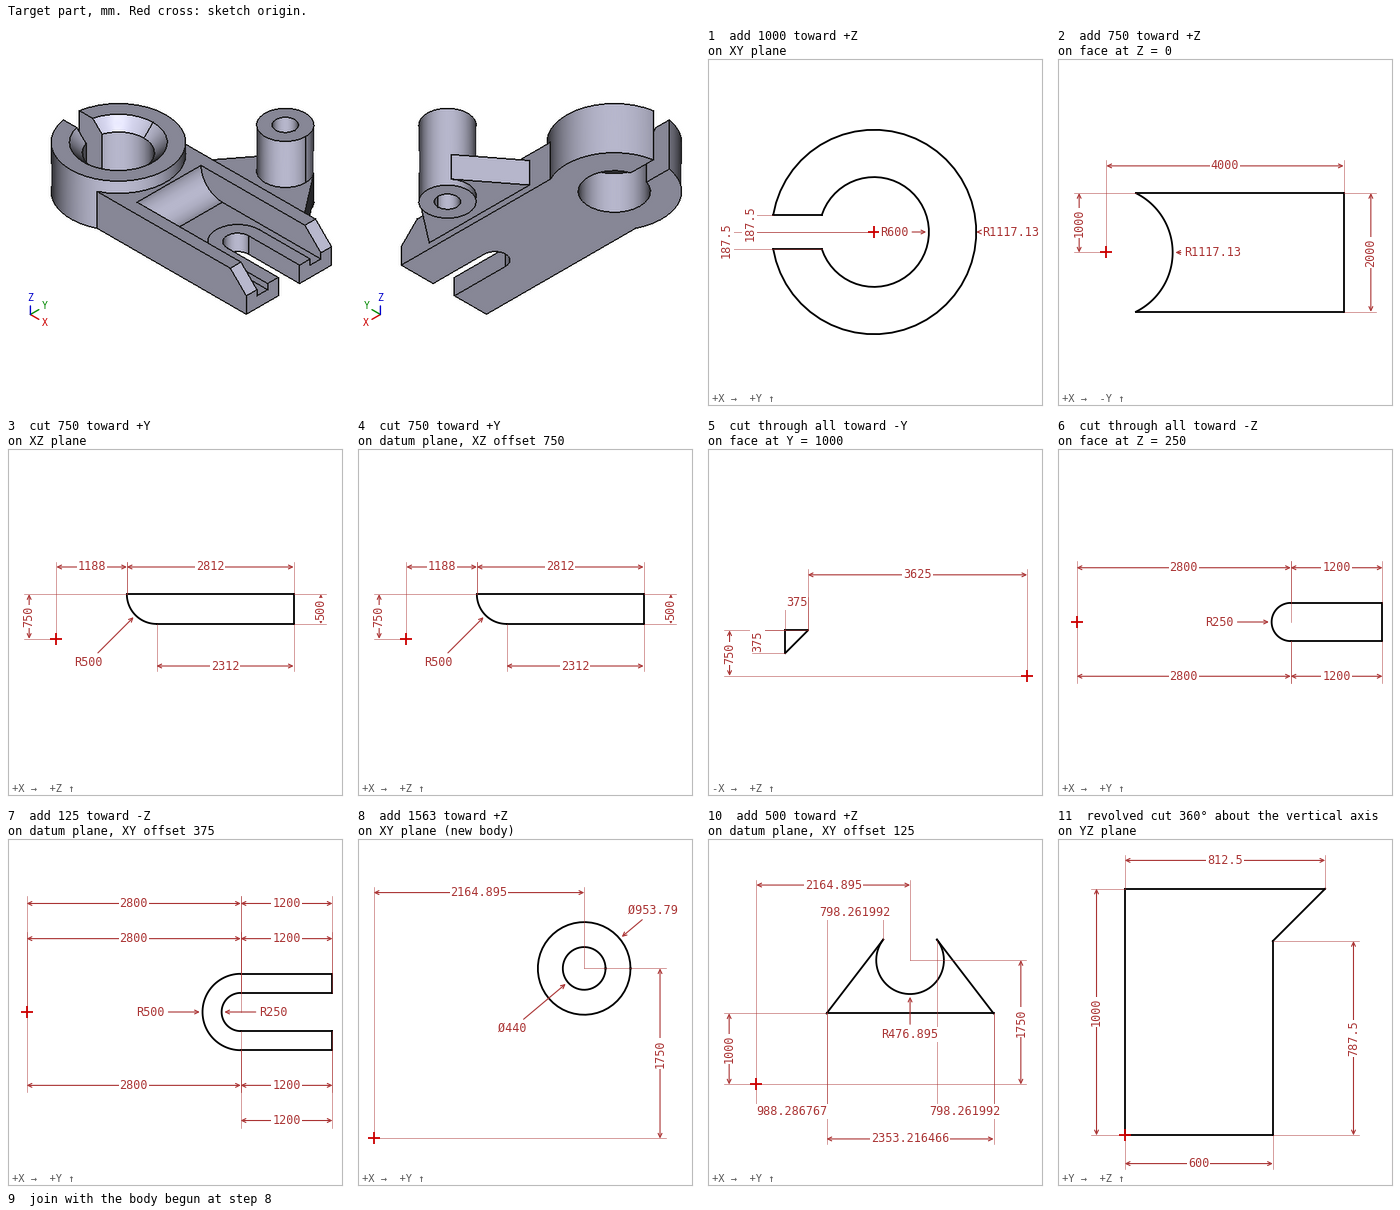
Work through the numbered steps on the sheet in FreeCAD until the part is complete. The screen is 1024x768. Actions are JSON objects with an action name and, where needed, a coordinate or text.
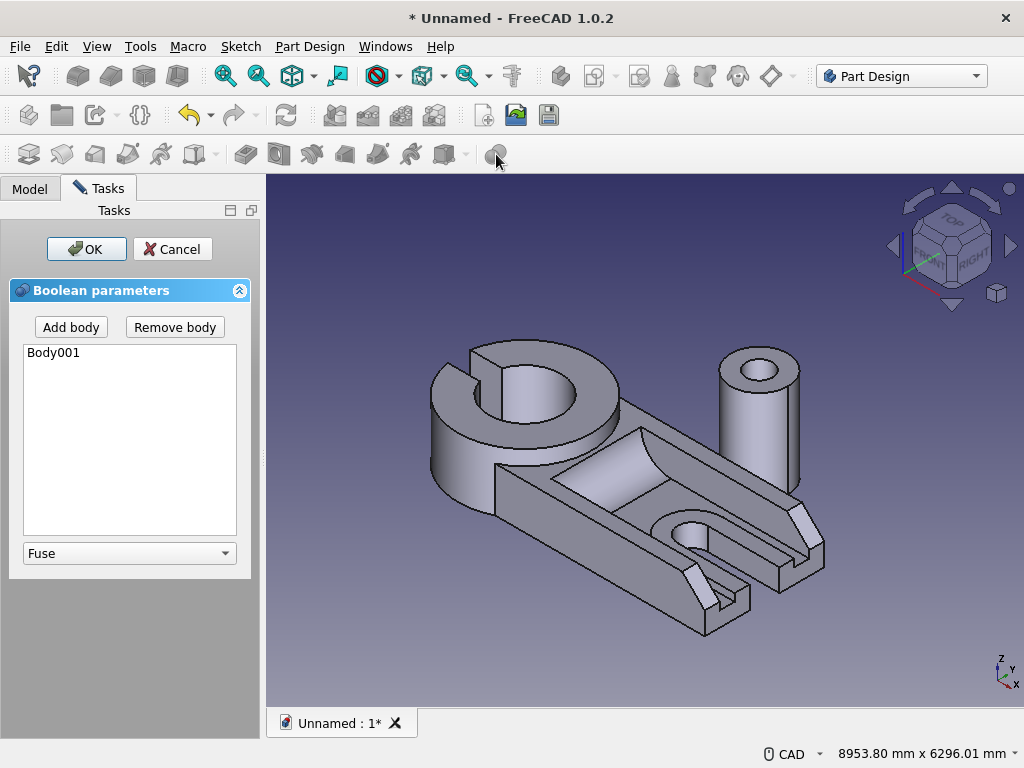
{"action": "left_click", "coordinate": [87, 249]}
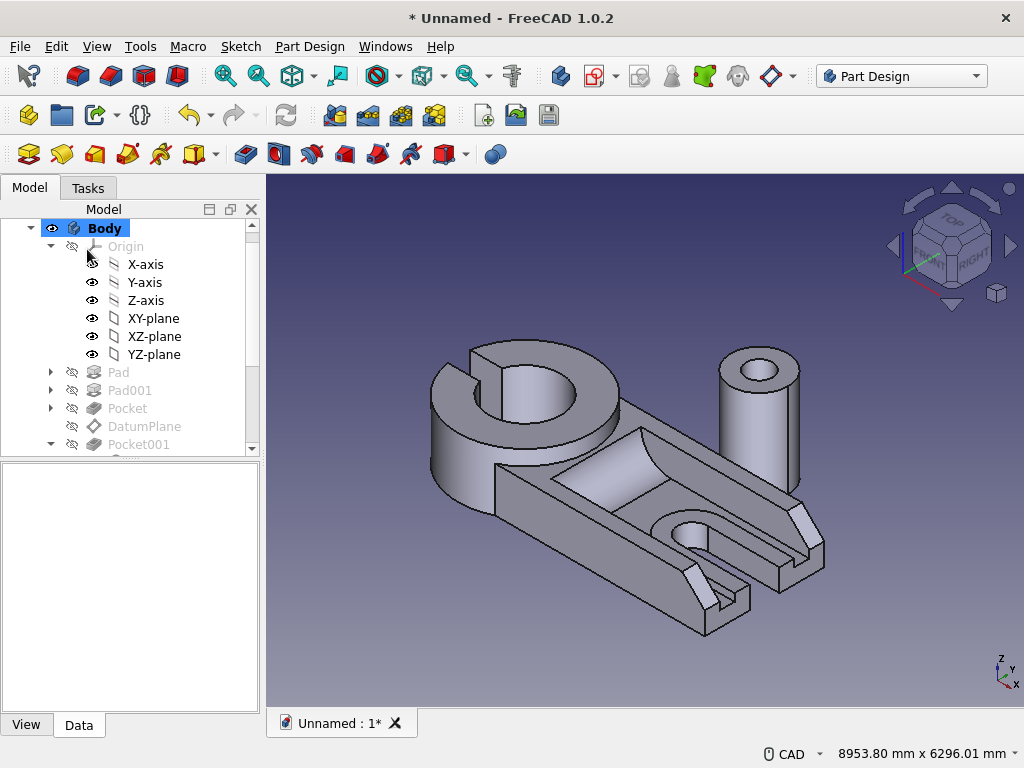
{"action": "left_click", "coordinate": [137, 318]}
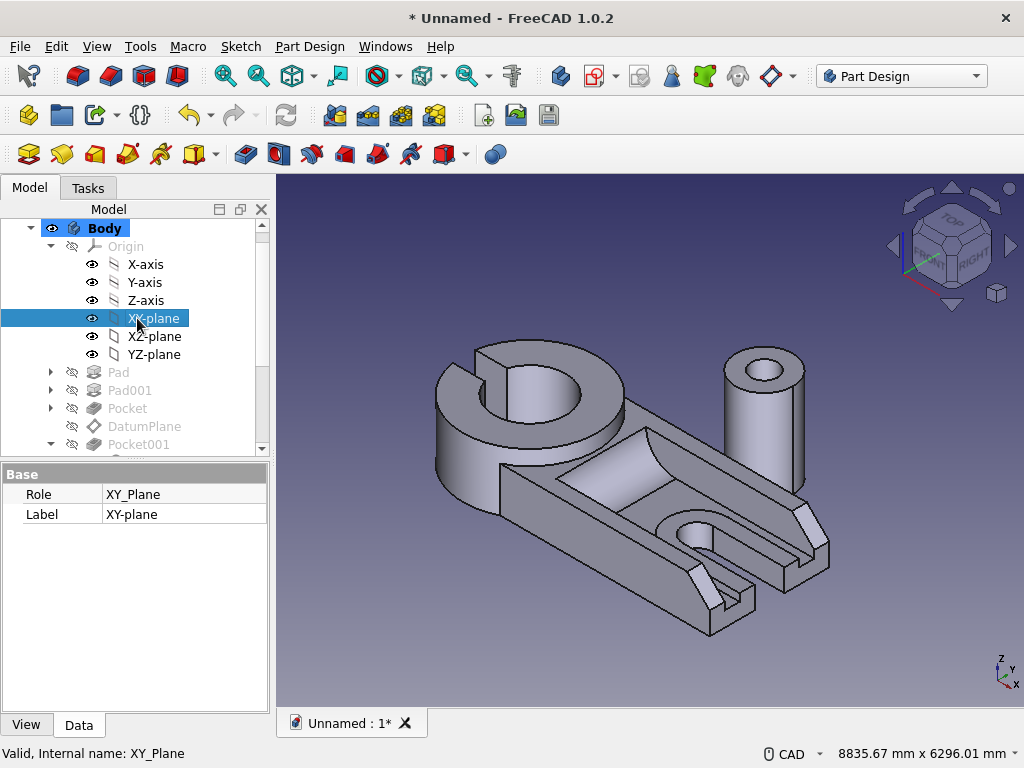
{"action": "left_click", "coordinate": [770, 76]}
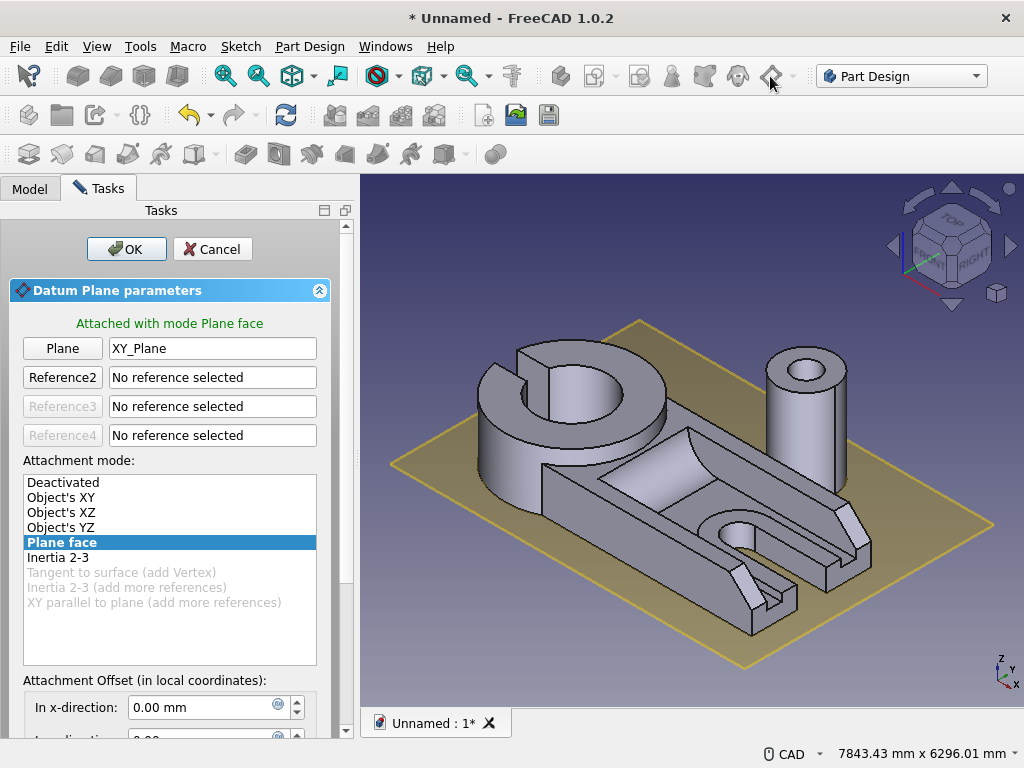
{"action": "scroll", "coordinate": [346, 479], "scroll_direction": "down", "scroll_amount": 2}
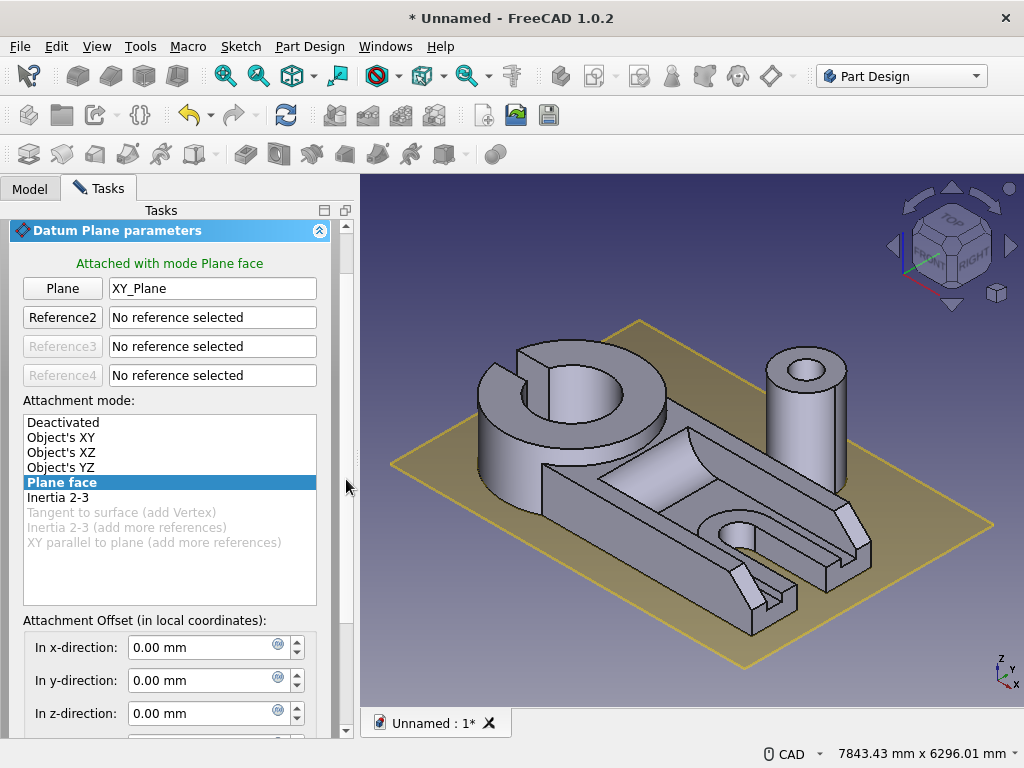
{"action": "triple_click", "coordinate": [210, 654]}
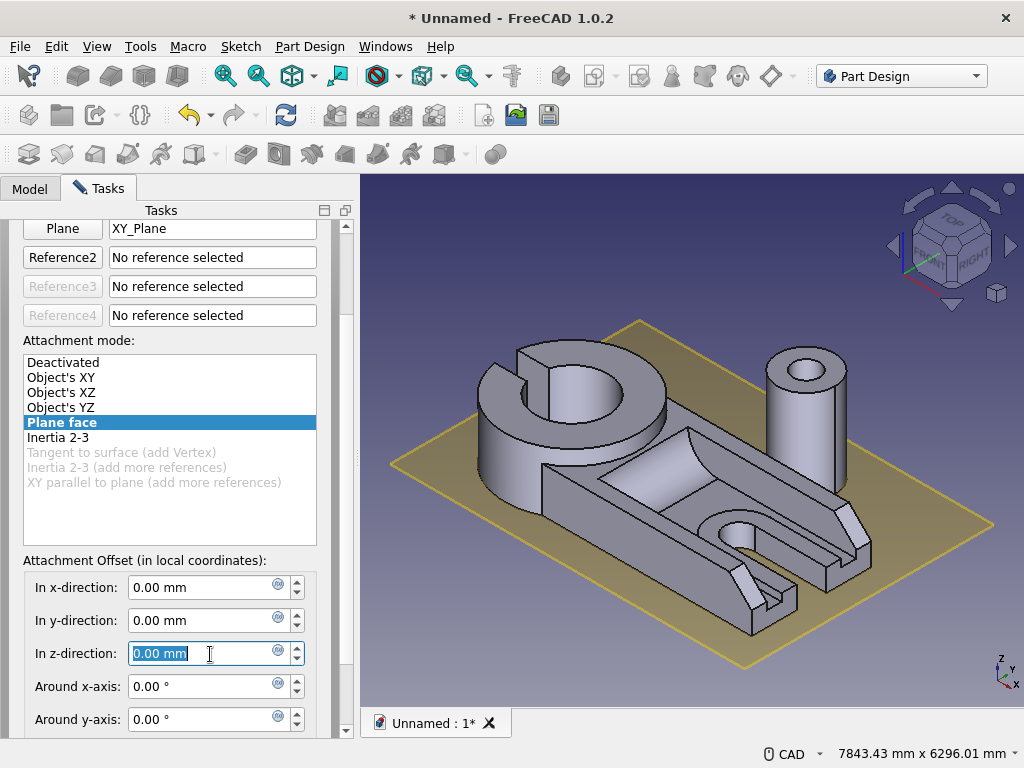
{"action": "type", "text": "125"}
{"action": "key", "text": "Tab"}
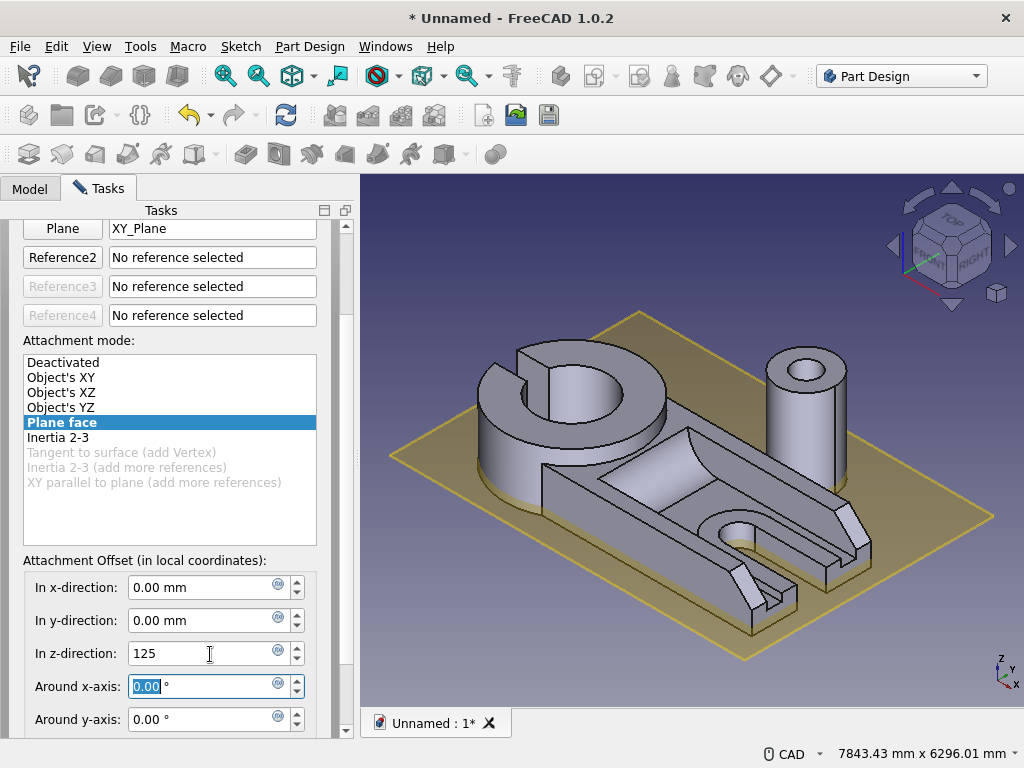
{"action": "scroll", "coordinate": [346, 479], "scroll_direction": "up", "scroll_amount": 3}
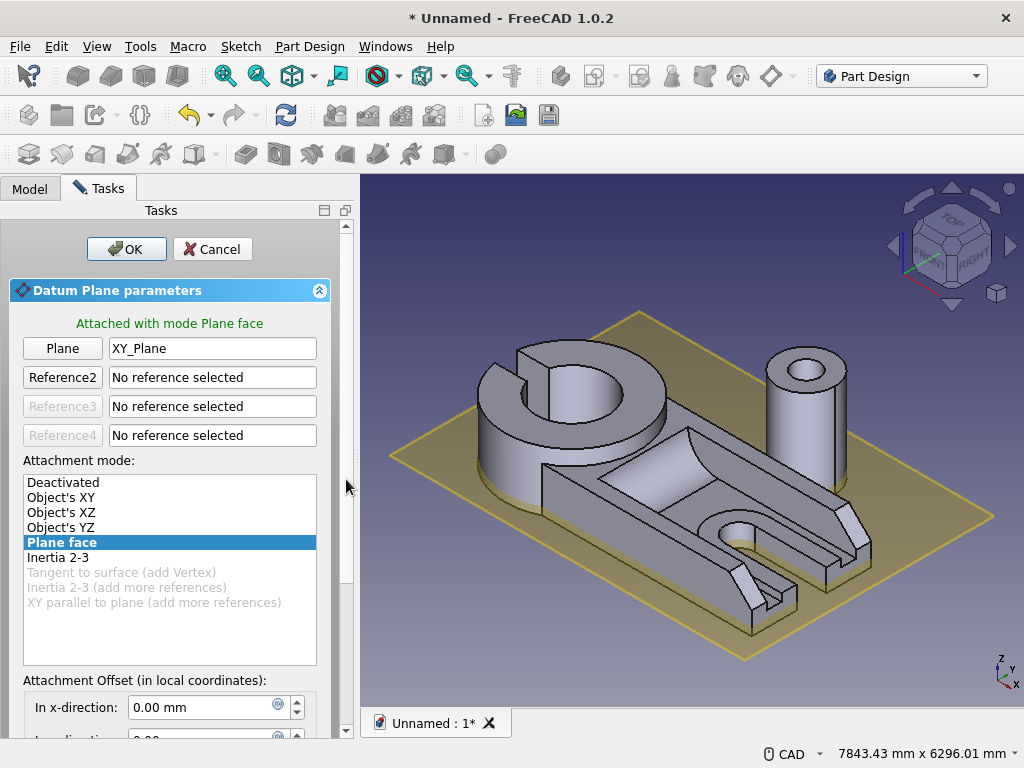
{"action": "left_click", "coordinate": [127, 249]}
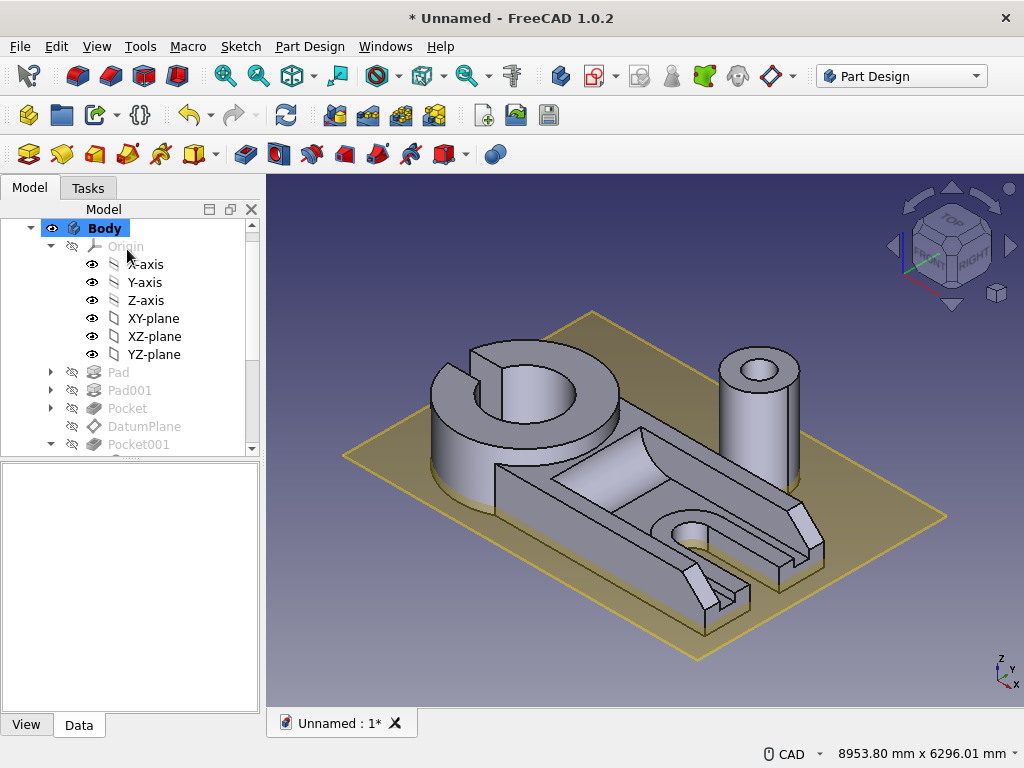
{"action": "scroll", "coordinate": [121, 332], "scroll_direction": "down", "scroll_amount": 3}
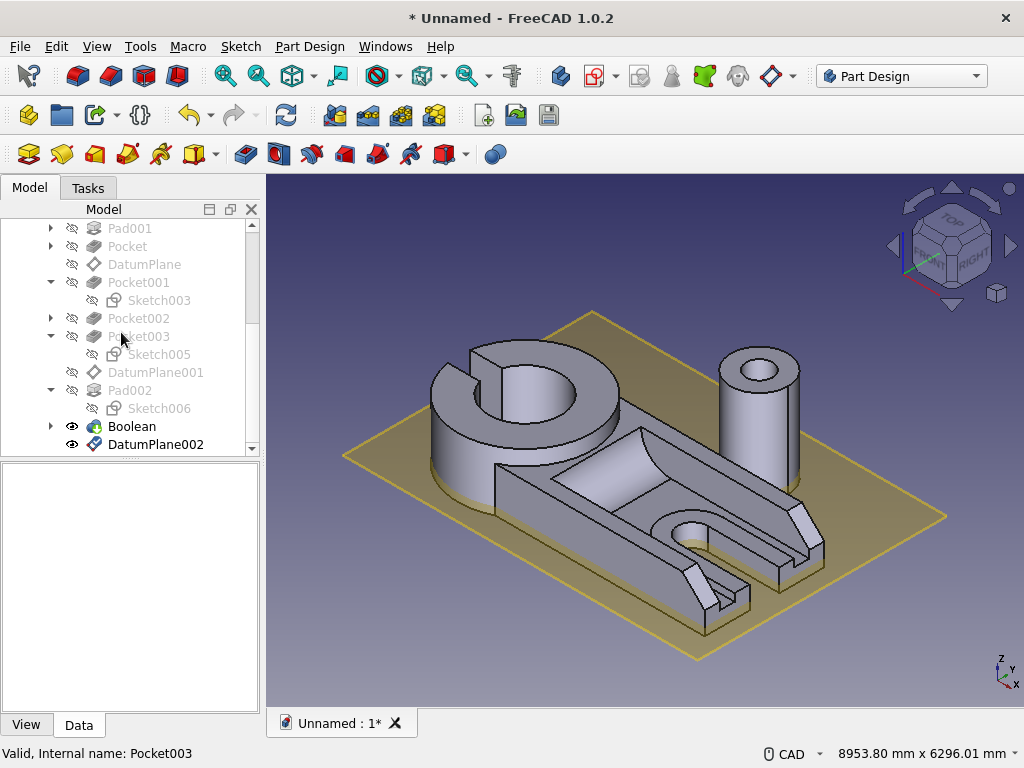
{"action": "left_click", "coordinate": [117, 444]}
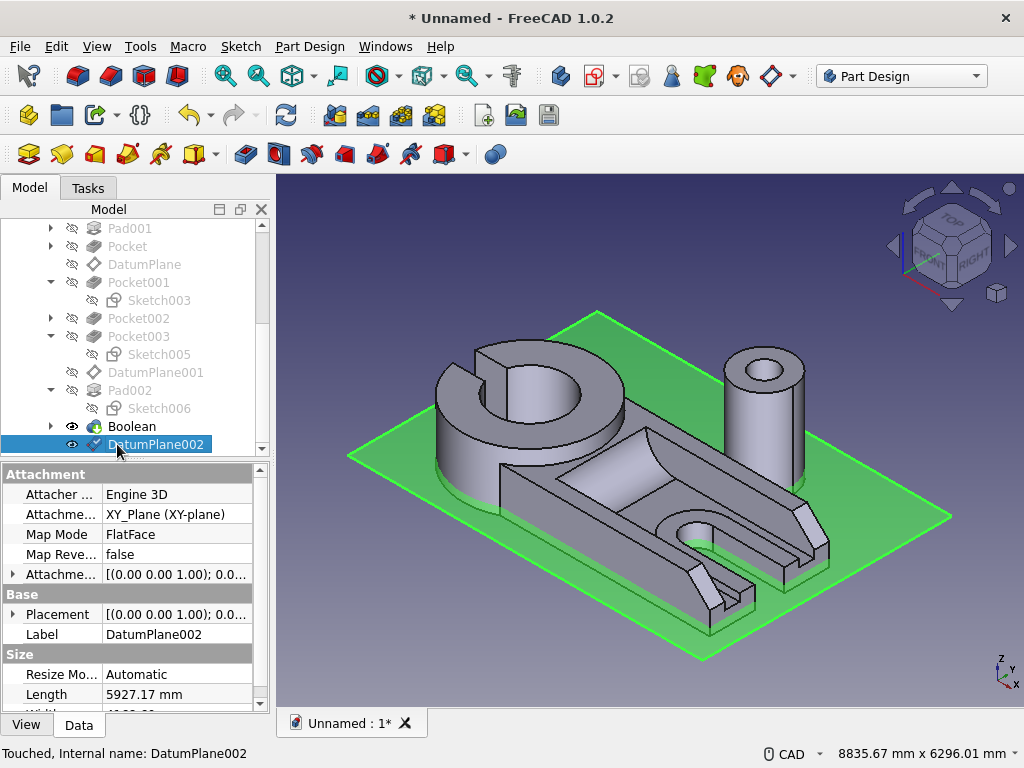
{"action": "left_click", "coordinate": [594, 76]}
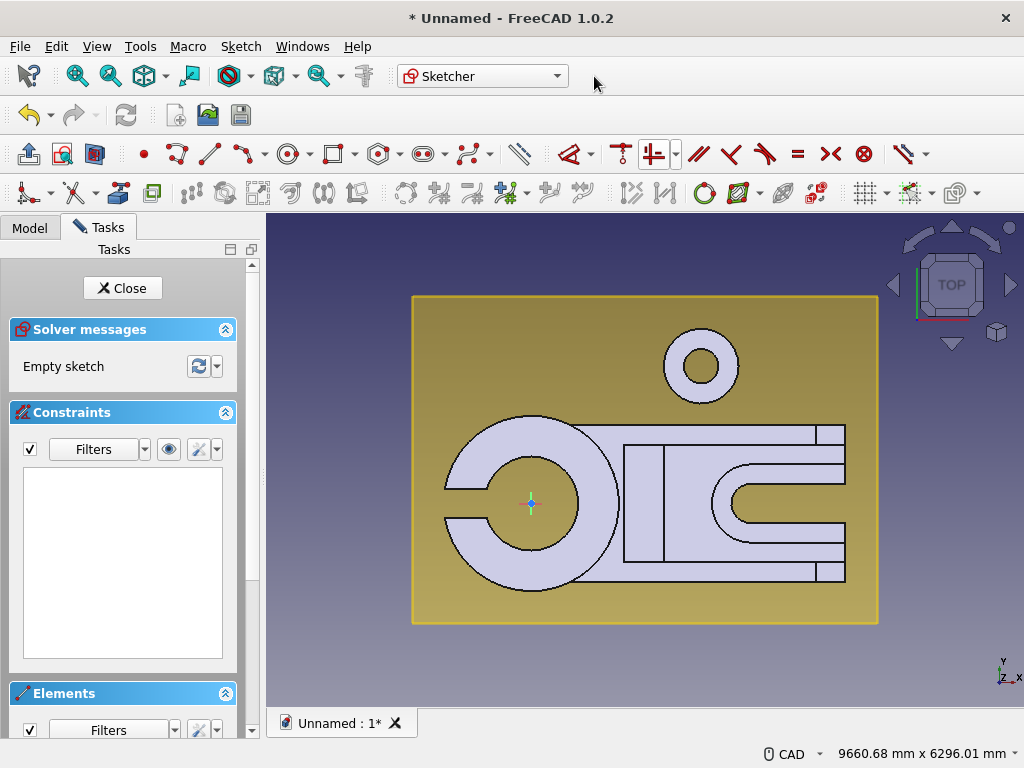
{"action": "key", "text": "q s"}